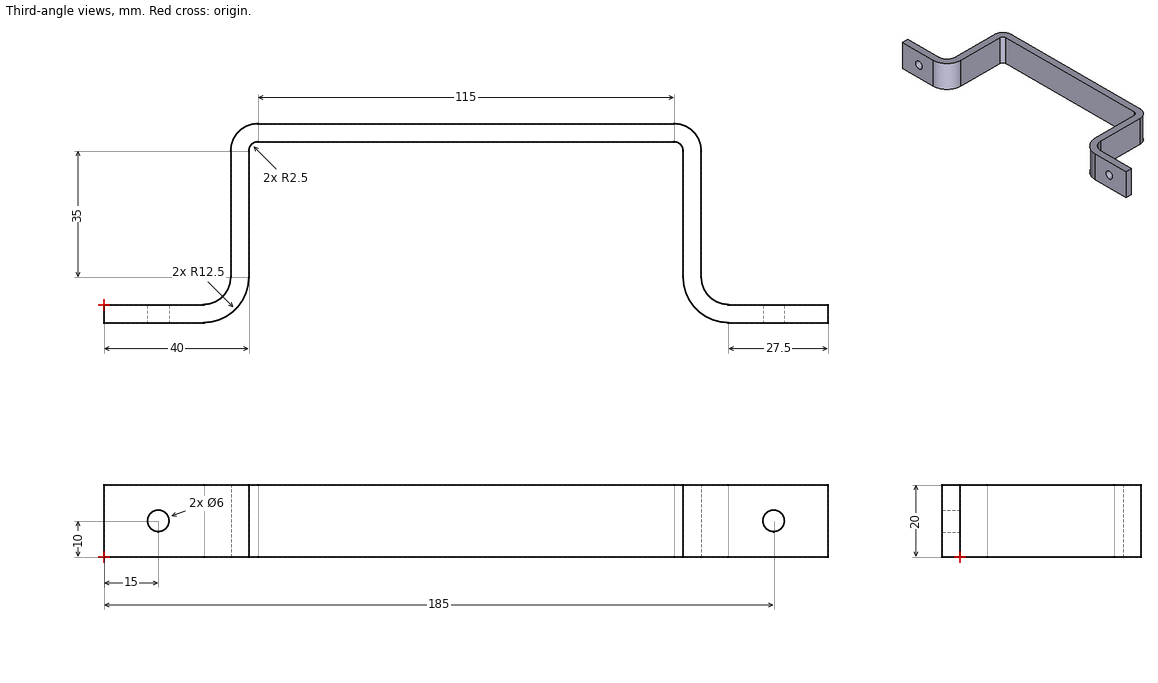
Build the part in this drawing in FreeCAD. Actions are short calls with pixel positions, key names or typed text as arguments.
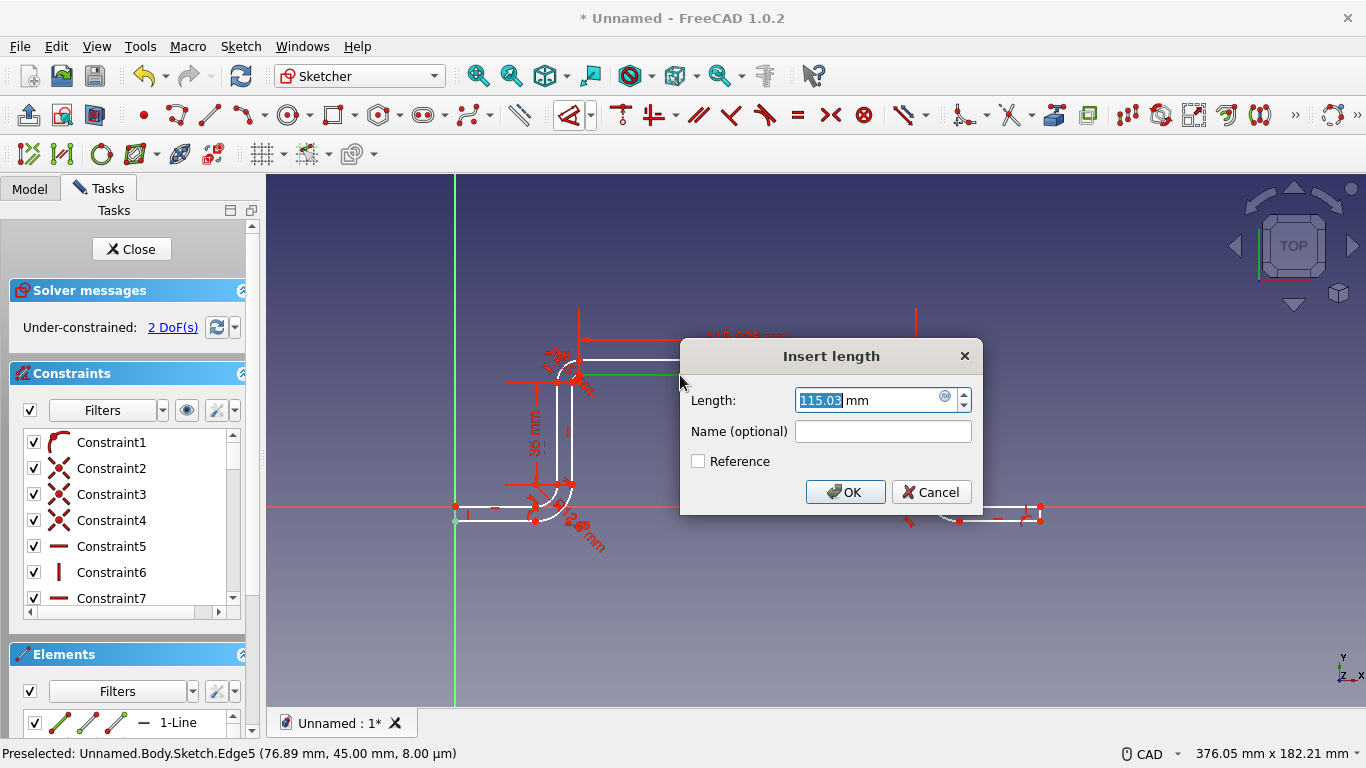
text(115)
key(Return)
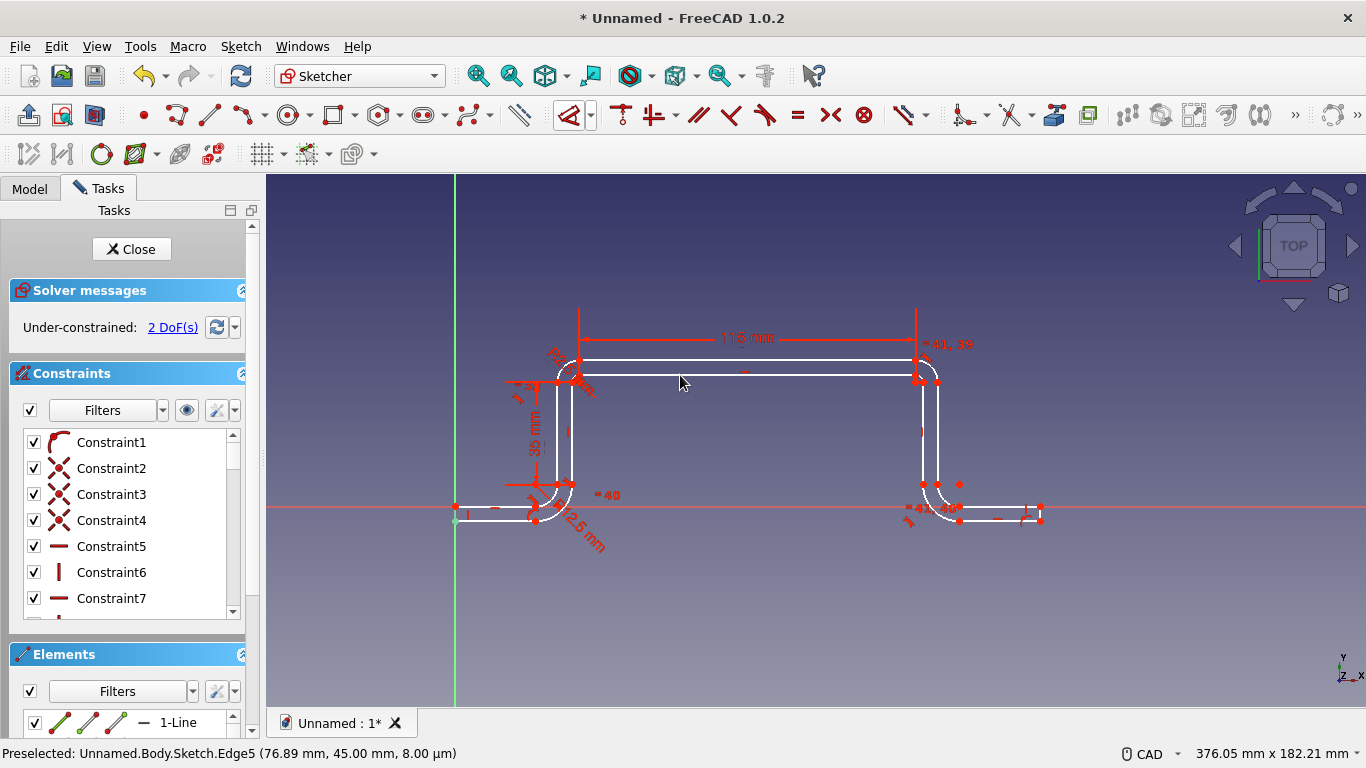
click(572, 485)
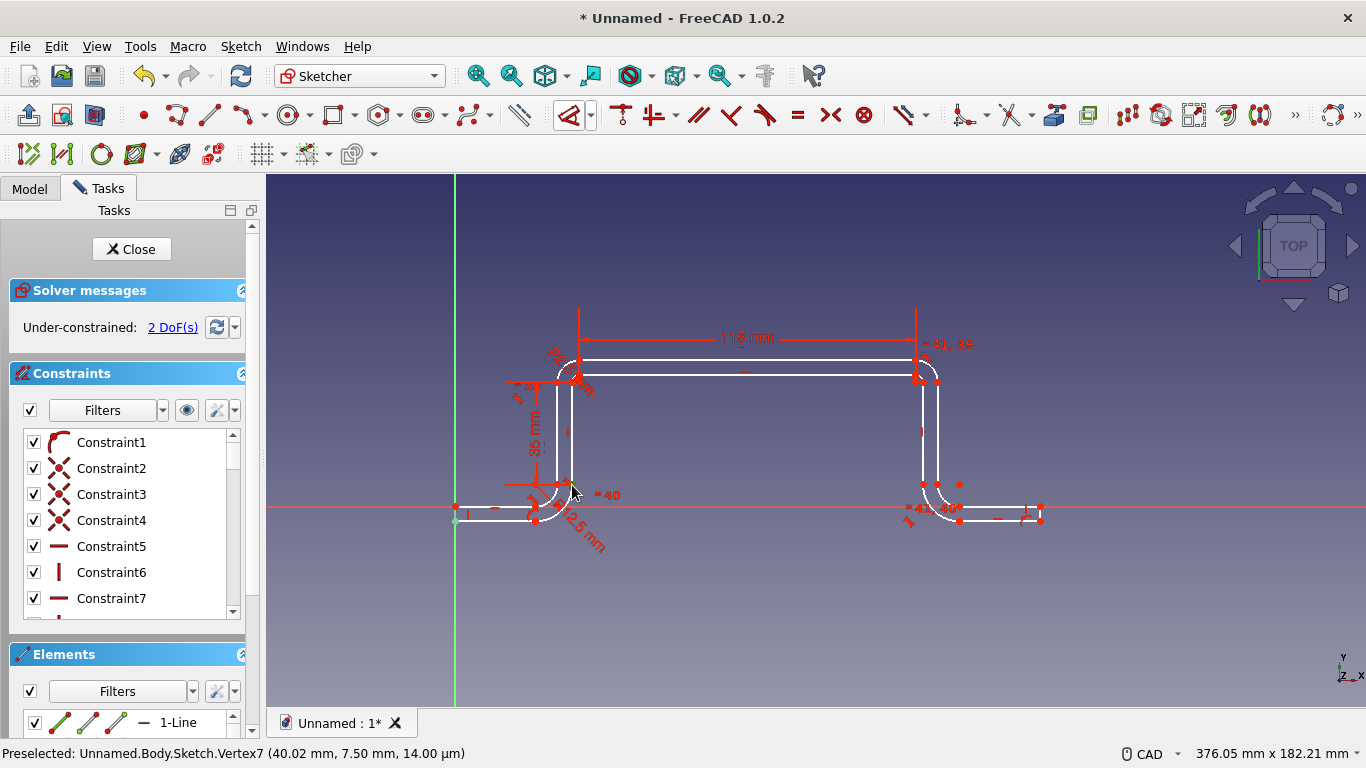
key(l)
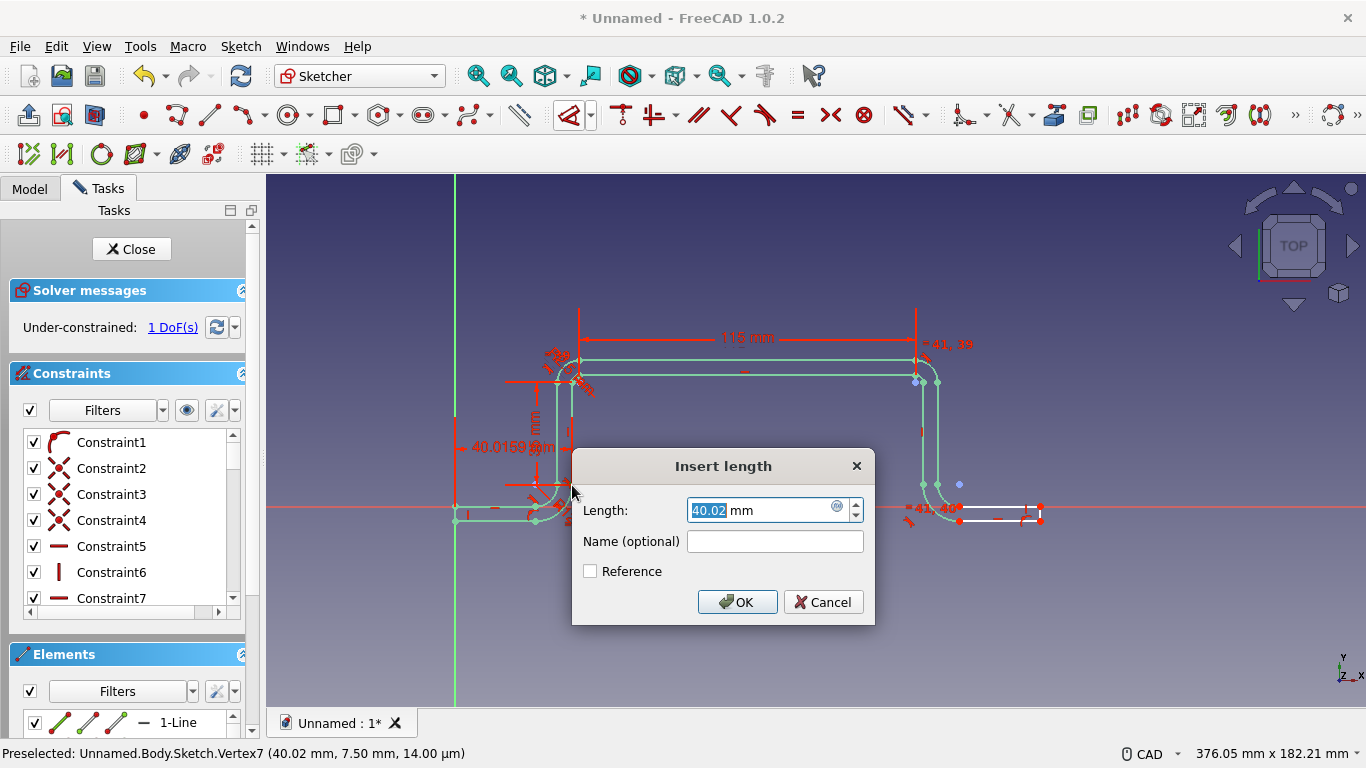
text(40)
key(Return)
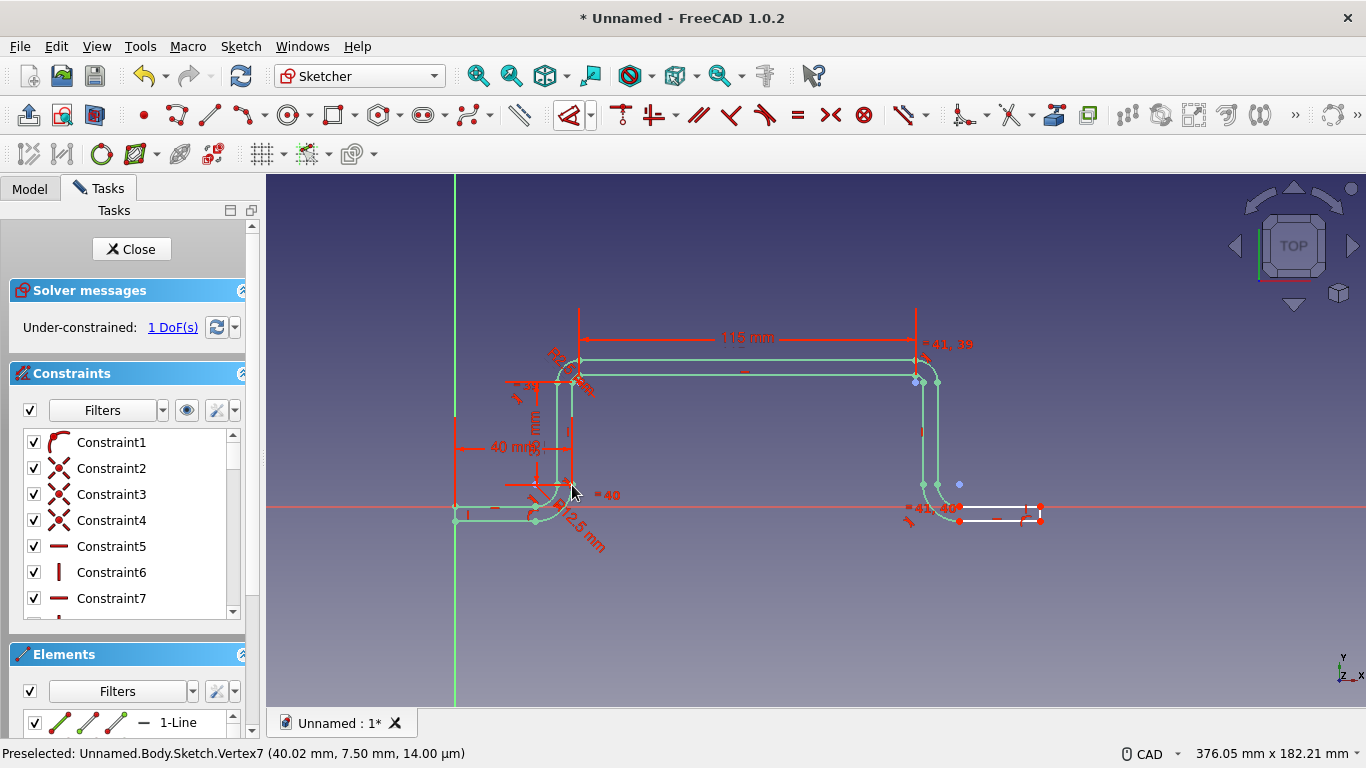
click(984, 521)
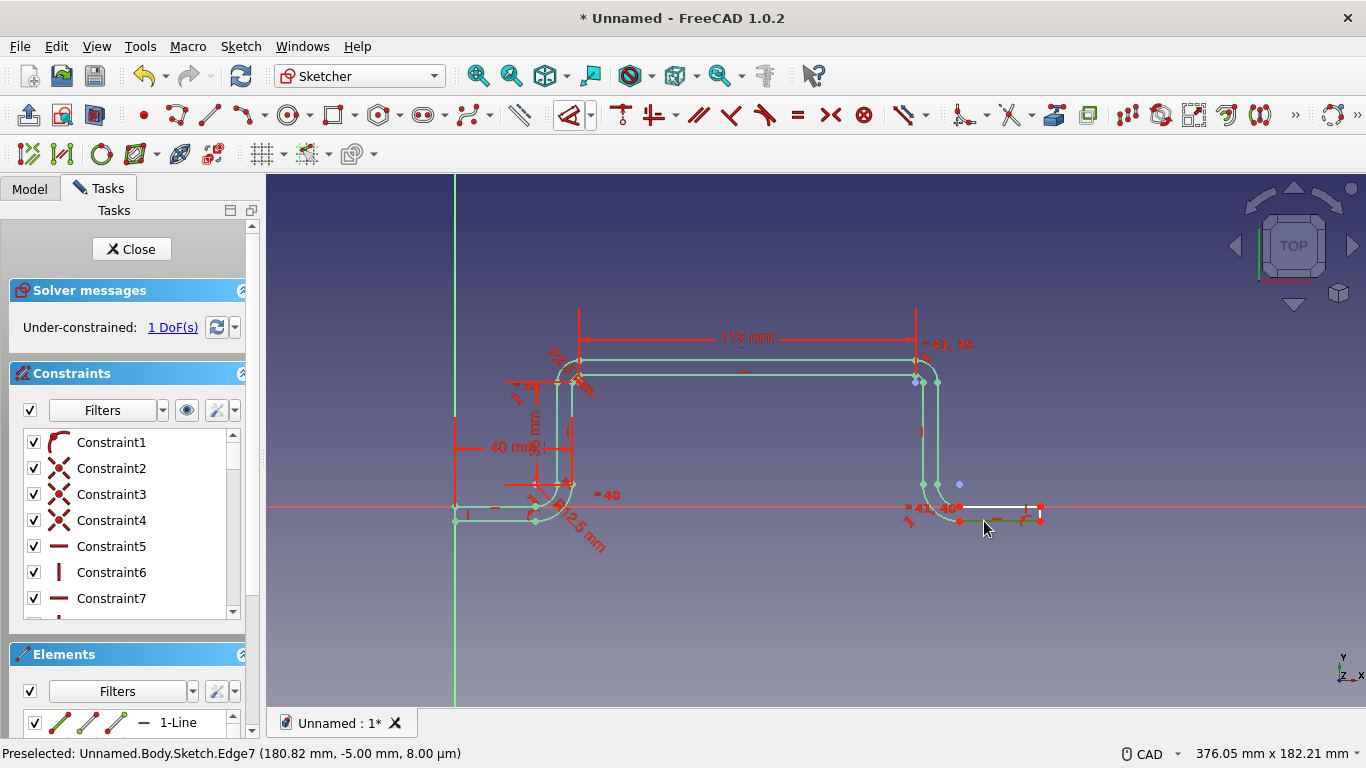
key(l)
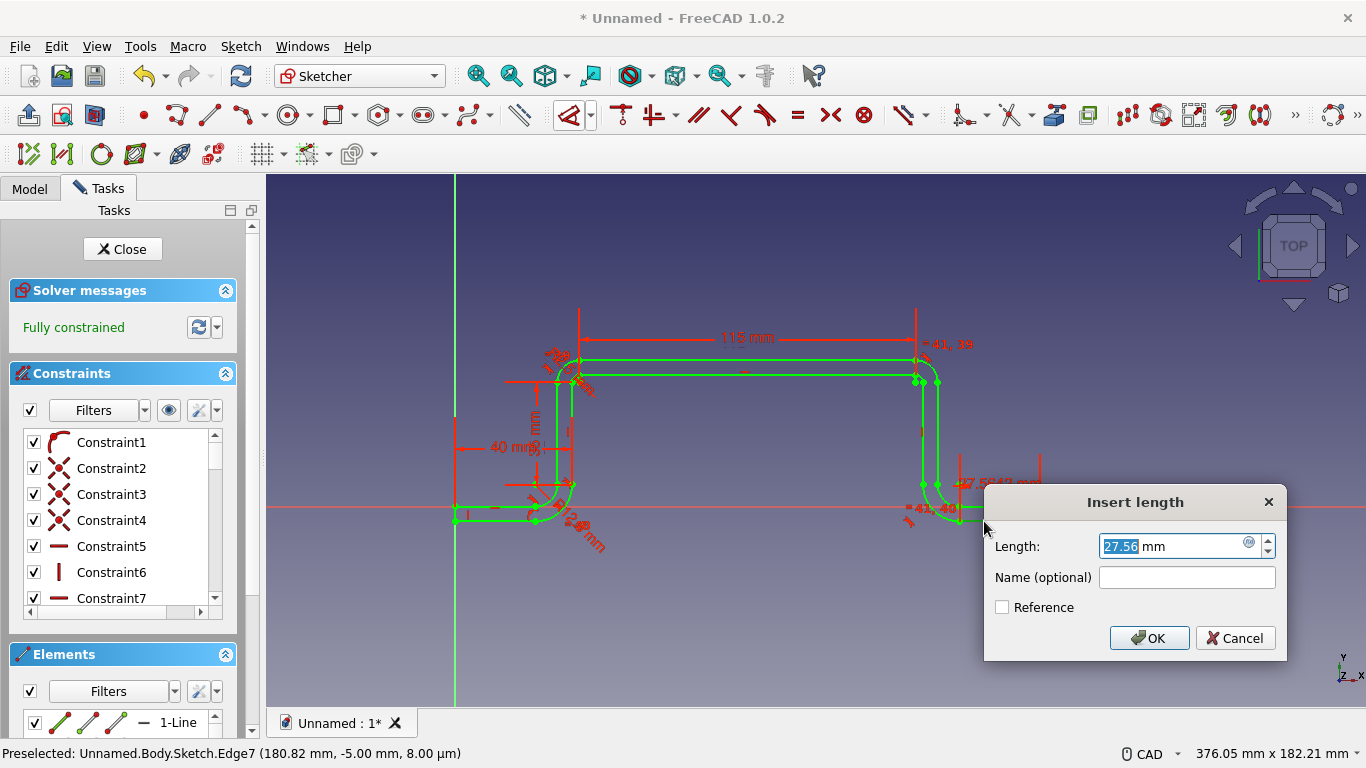
text(27.5)
key(Return)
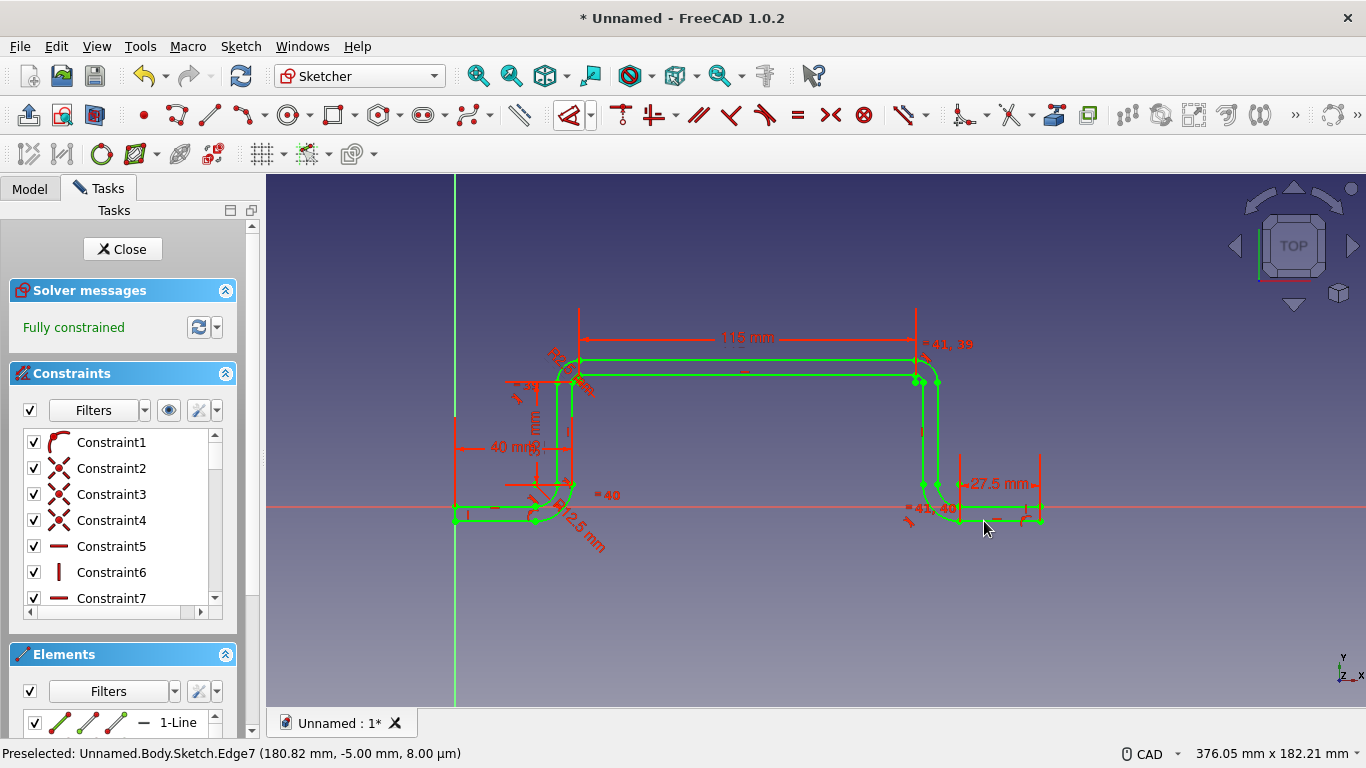
click(123, 249)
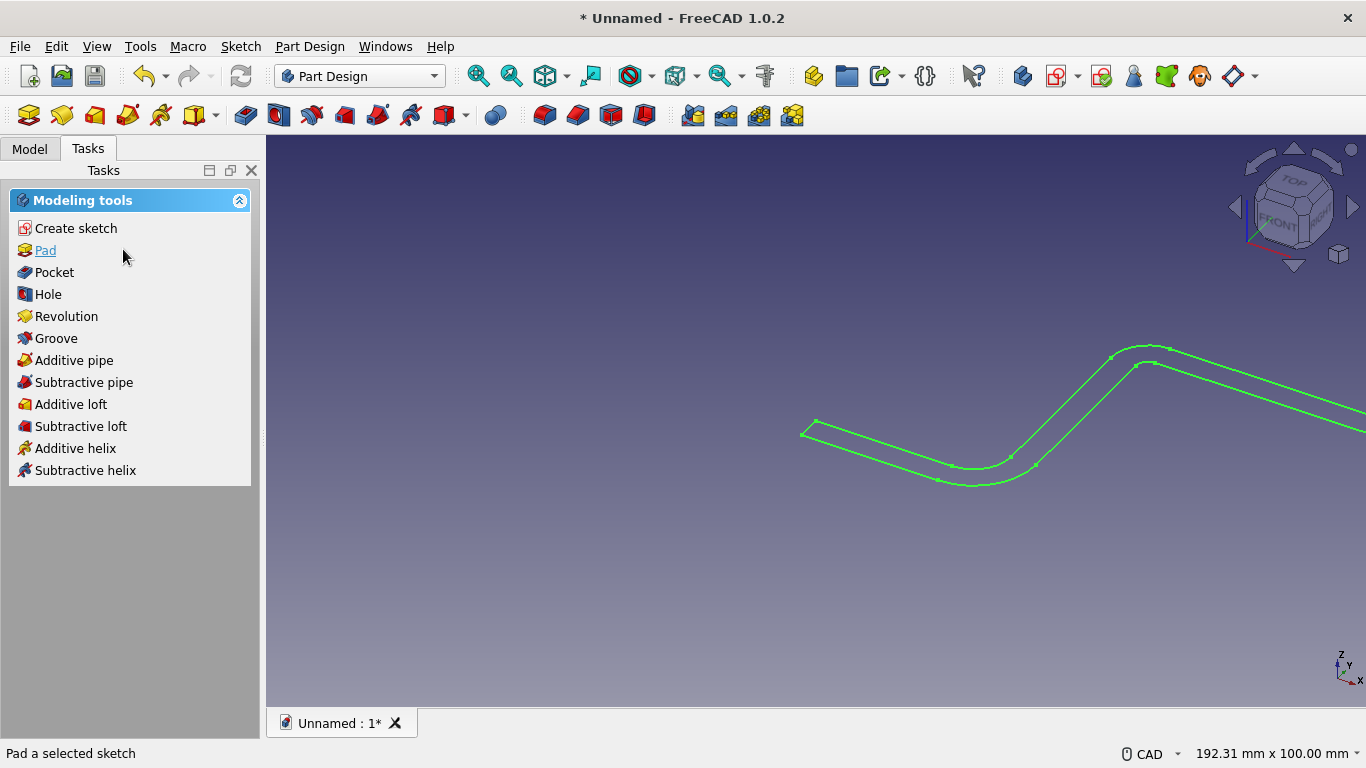
click(29, 116)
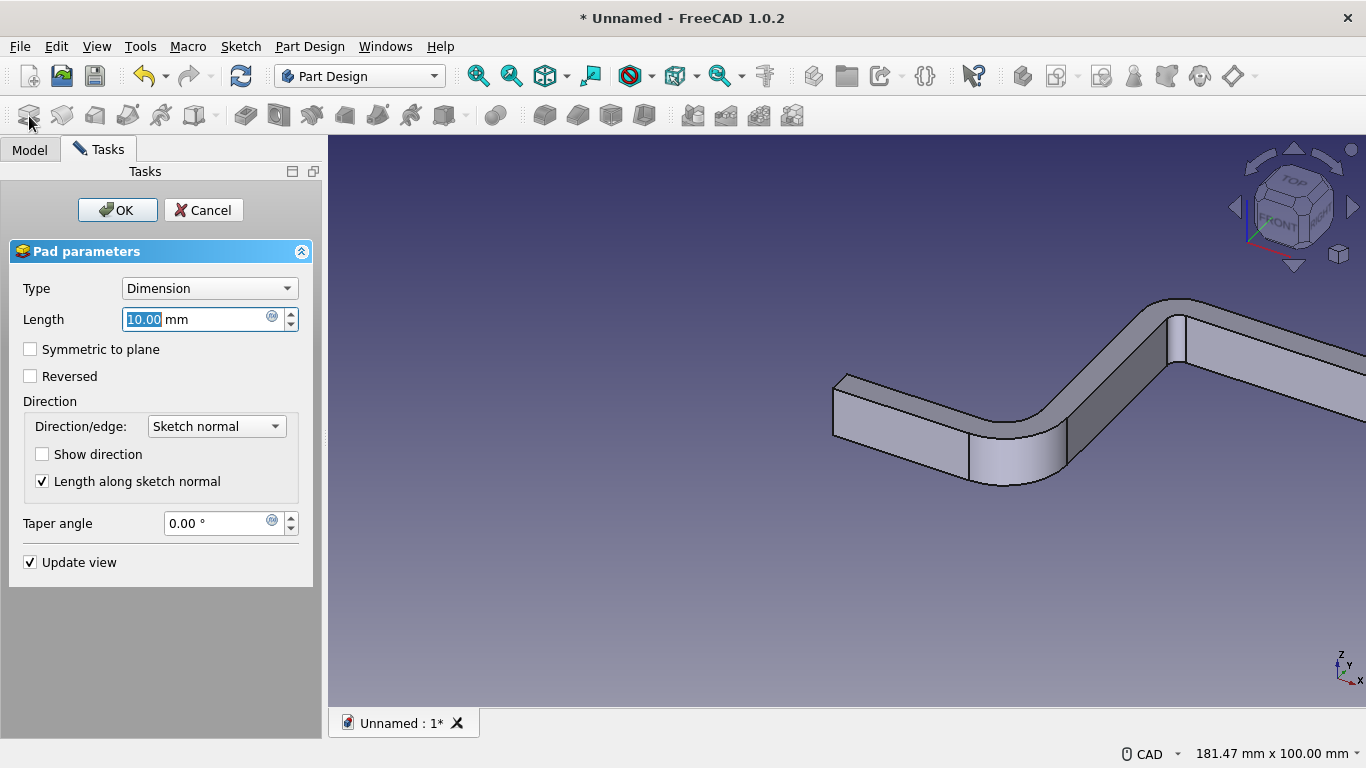
text(20)
key(Tab)